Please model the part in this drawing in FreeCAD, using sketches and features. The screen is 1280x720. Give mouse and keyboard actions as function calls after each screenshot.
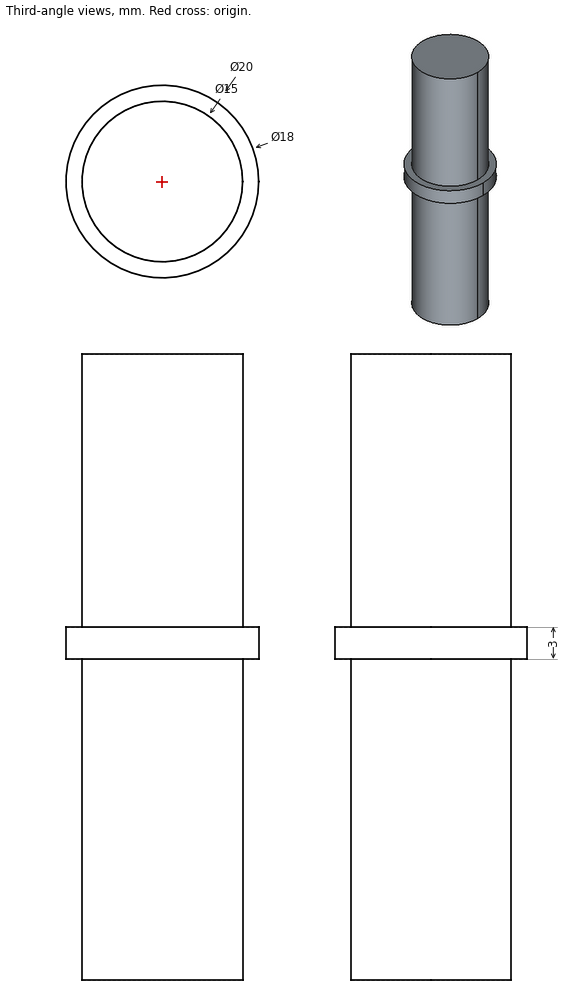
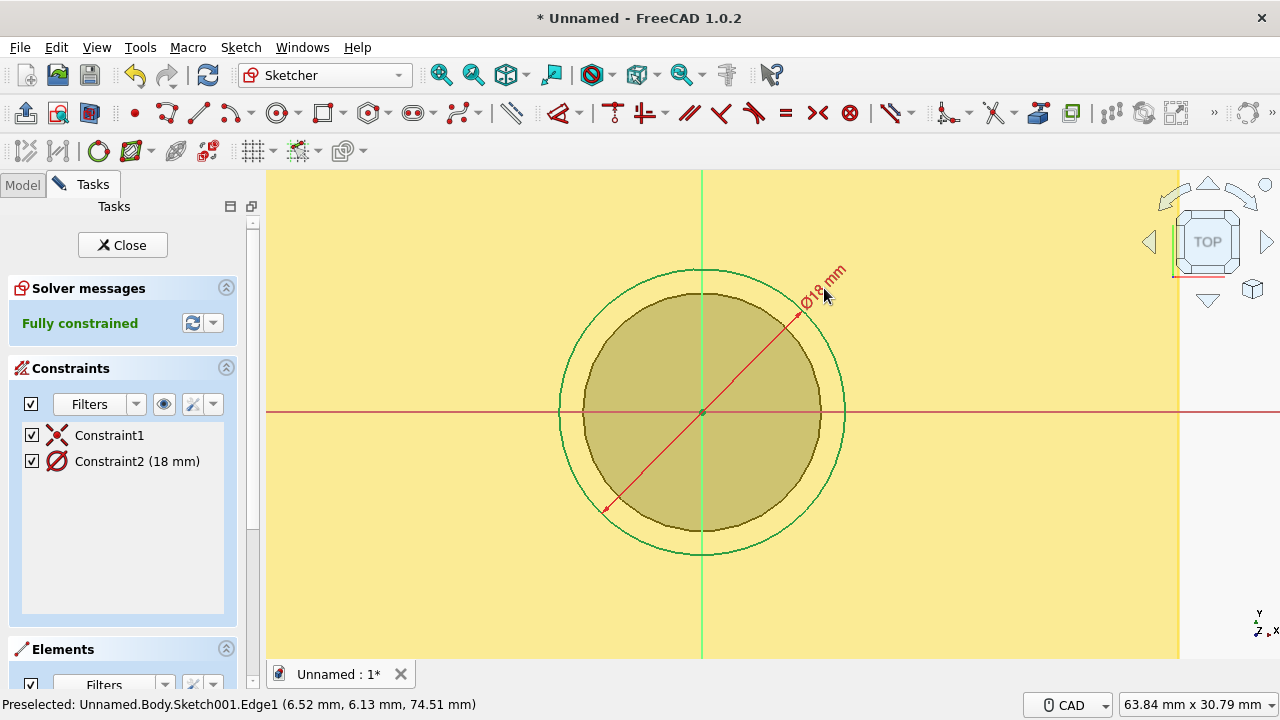
click(123, 245)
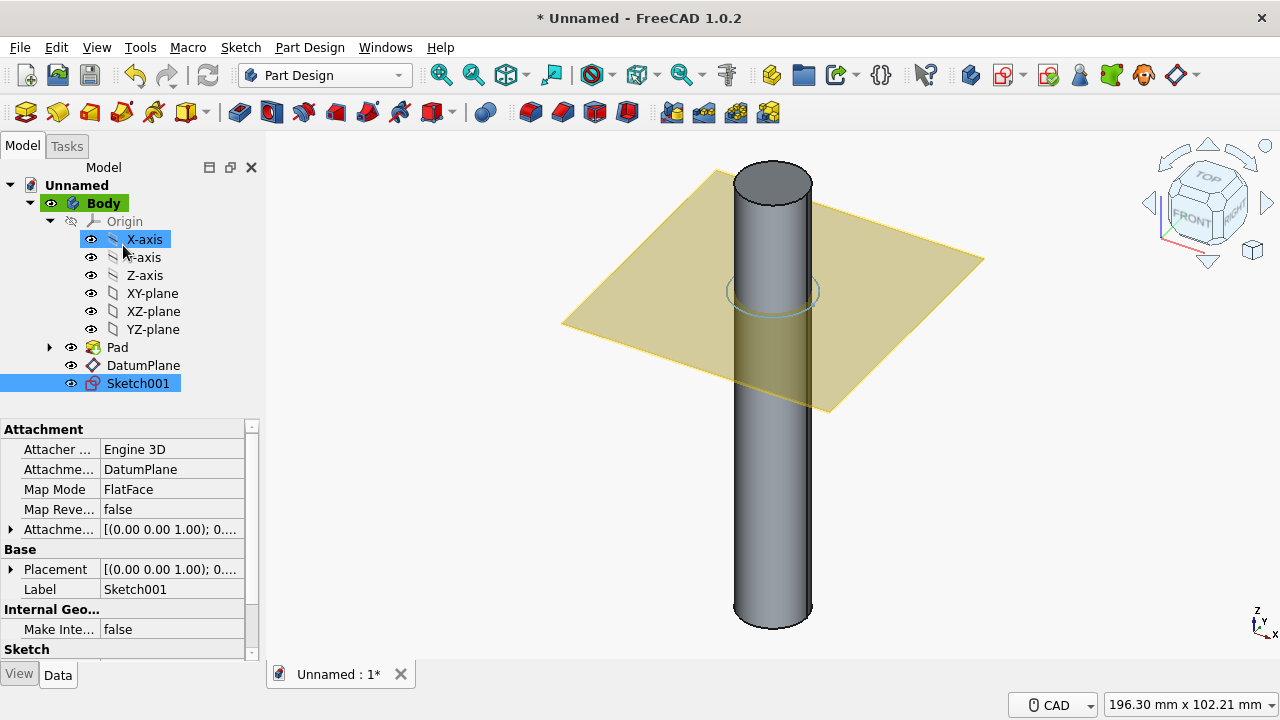
click(26, 112)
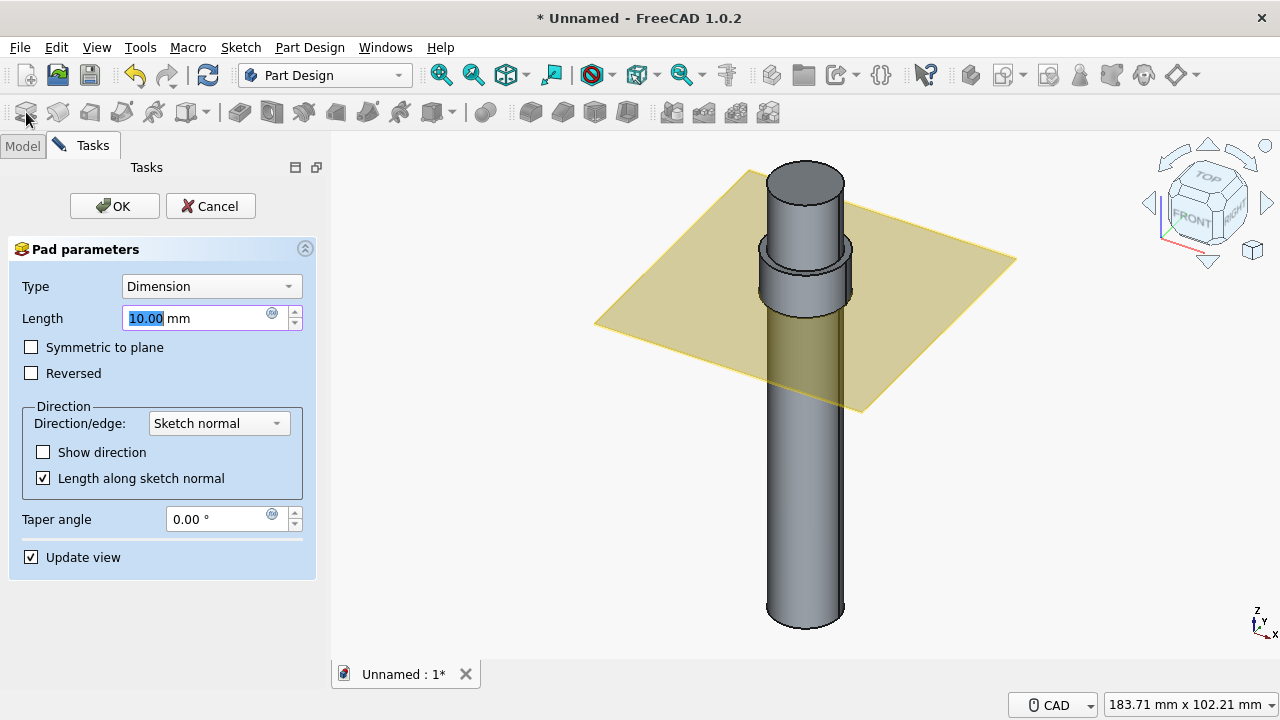
text(3)
key(Tab)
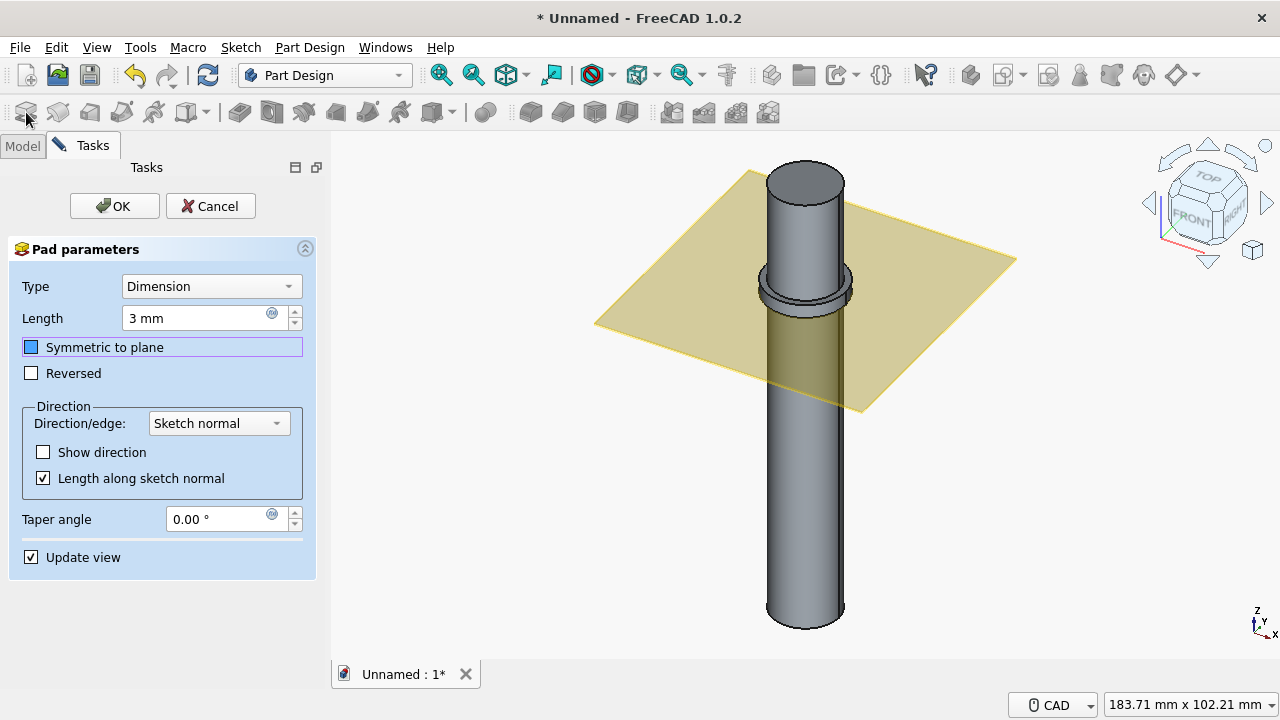
click(30, 373)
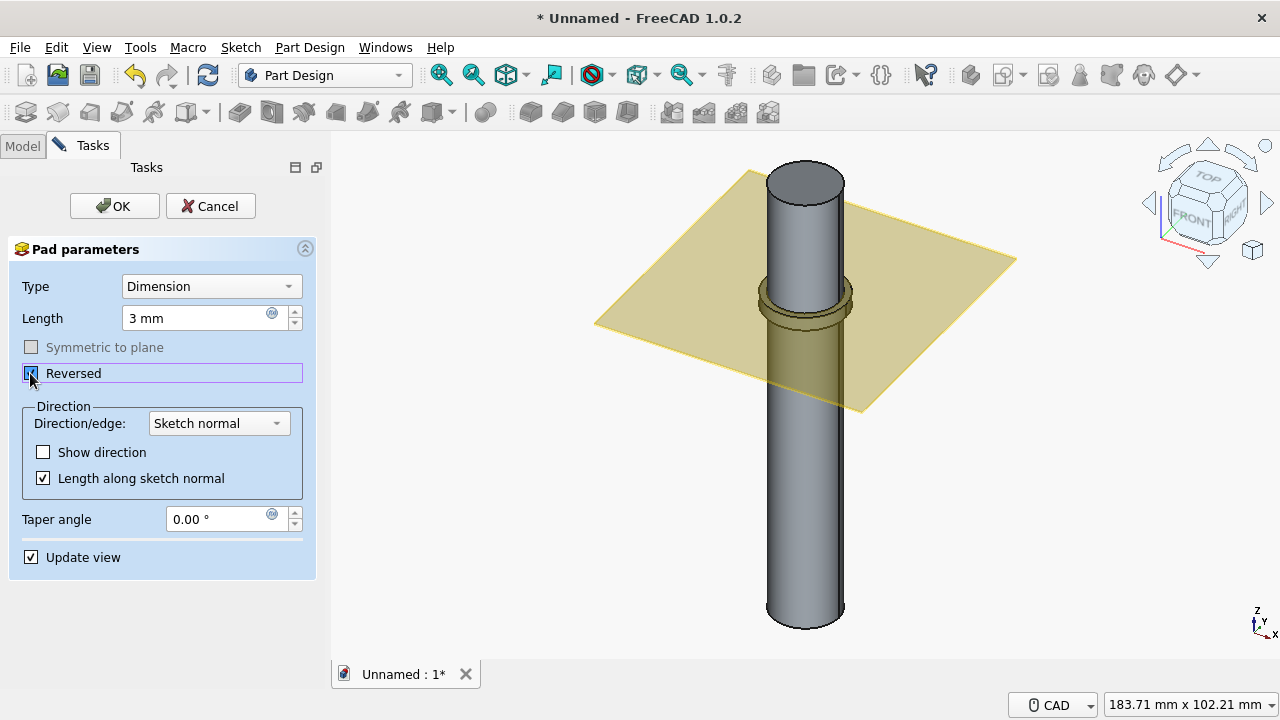
click(115, 206)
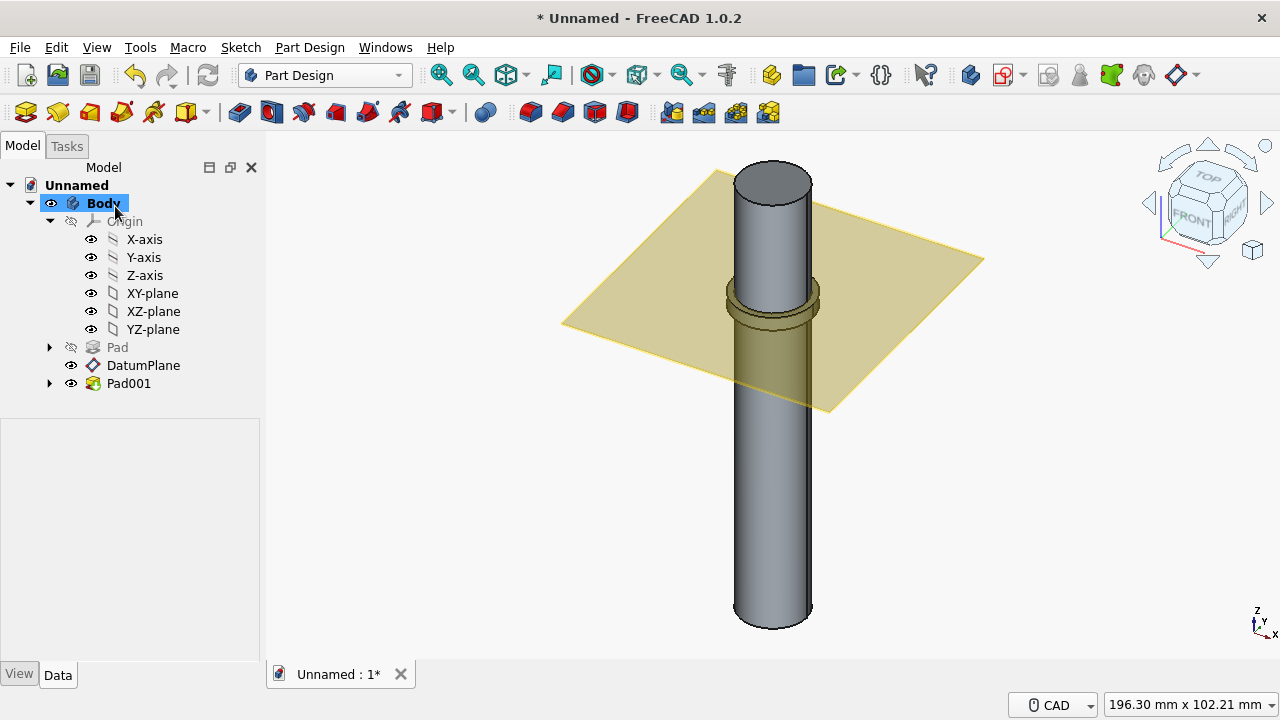
click(116, 365)
key(space)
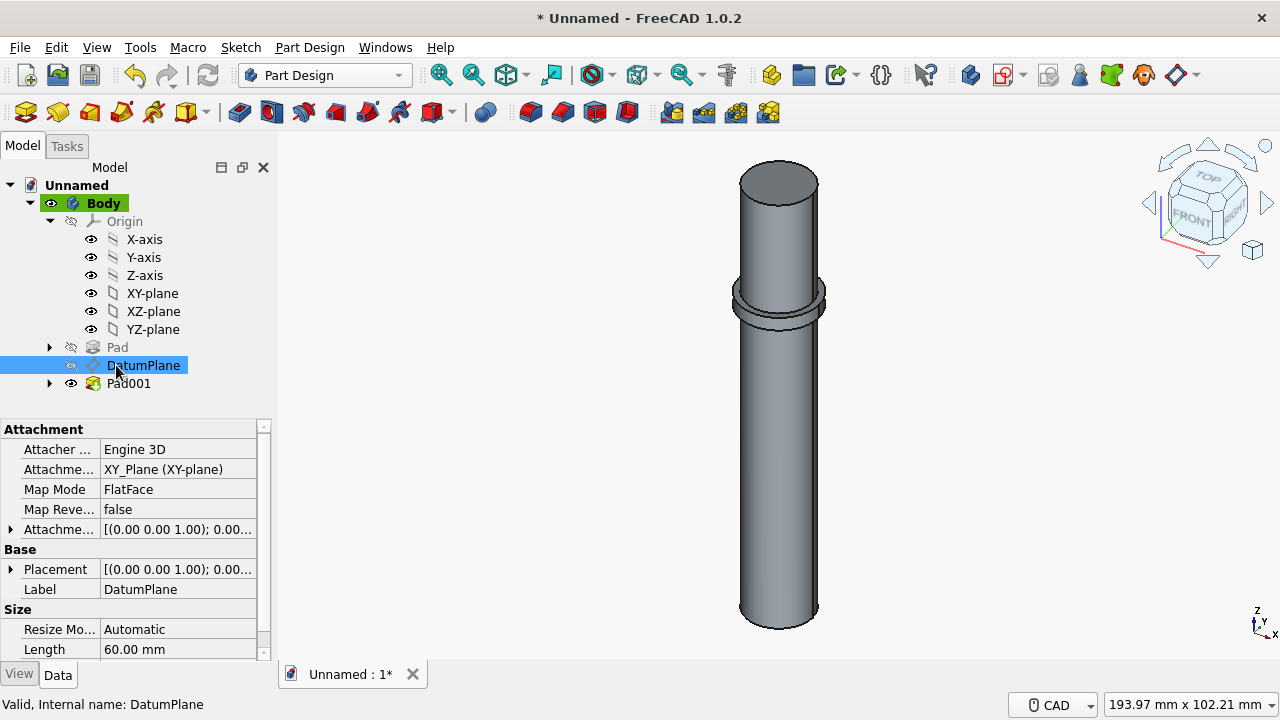
click(136, 293)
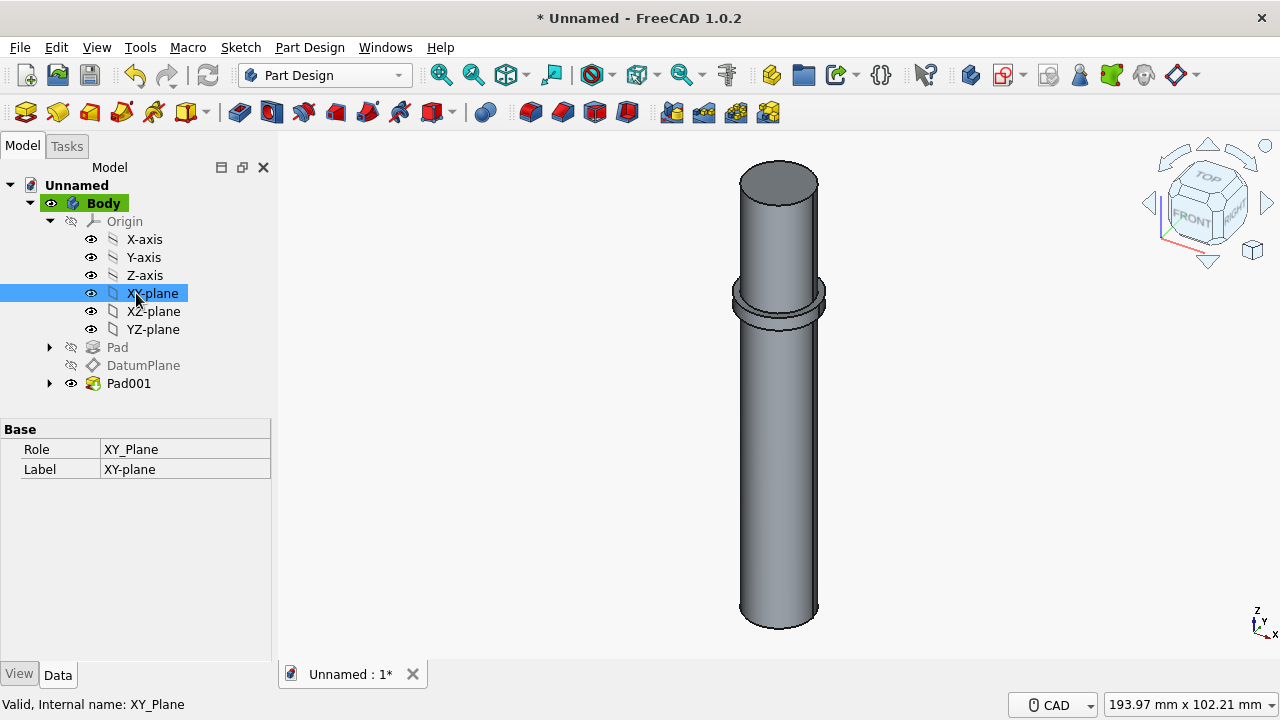
click(1176, 76)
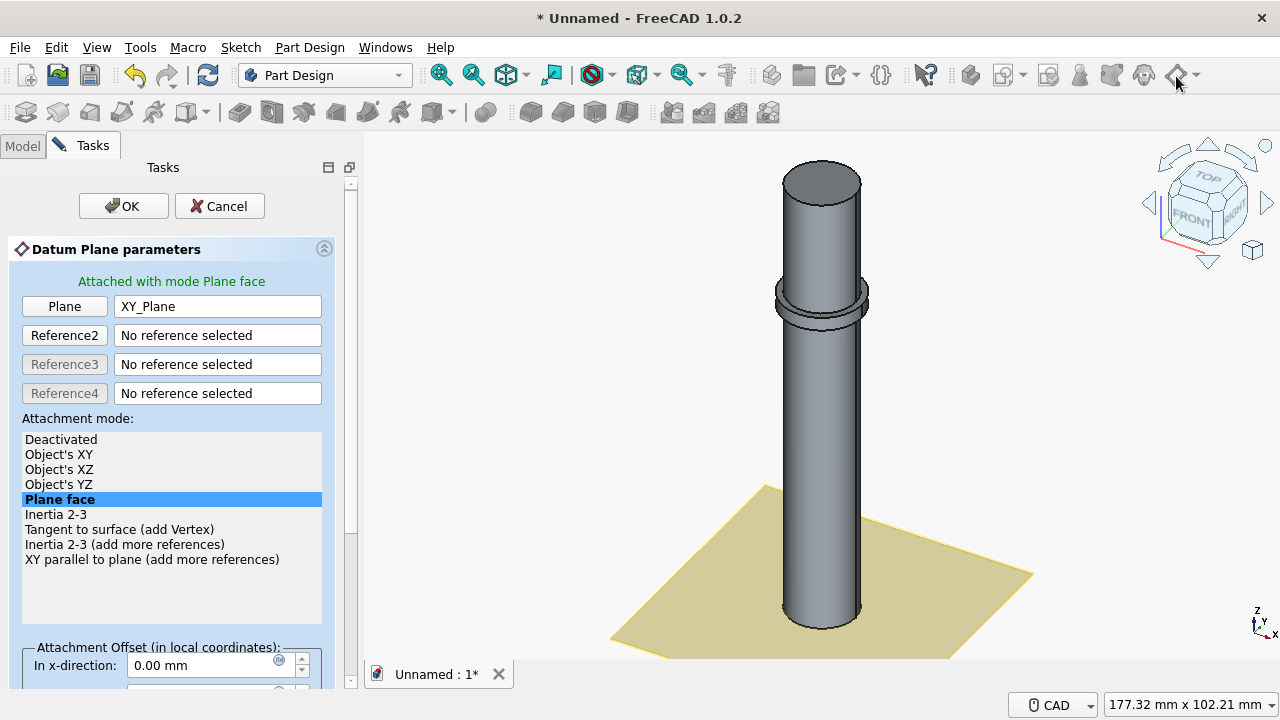
scroll(351, 432, down, 2)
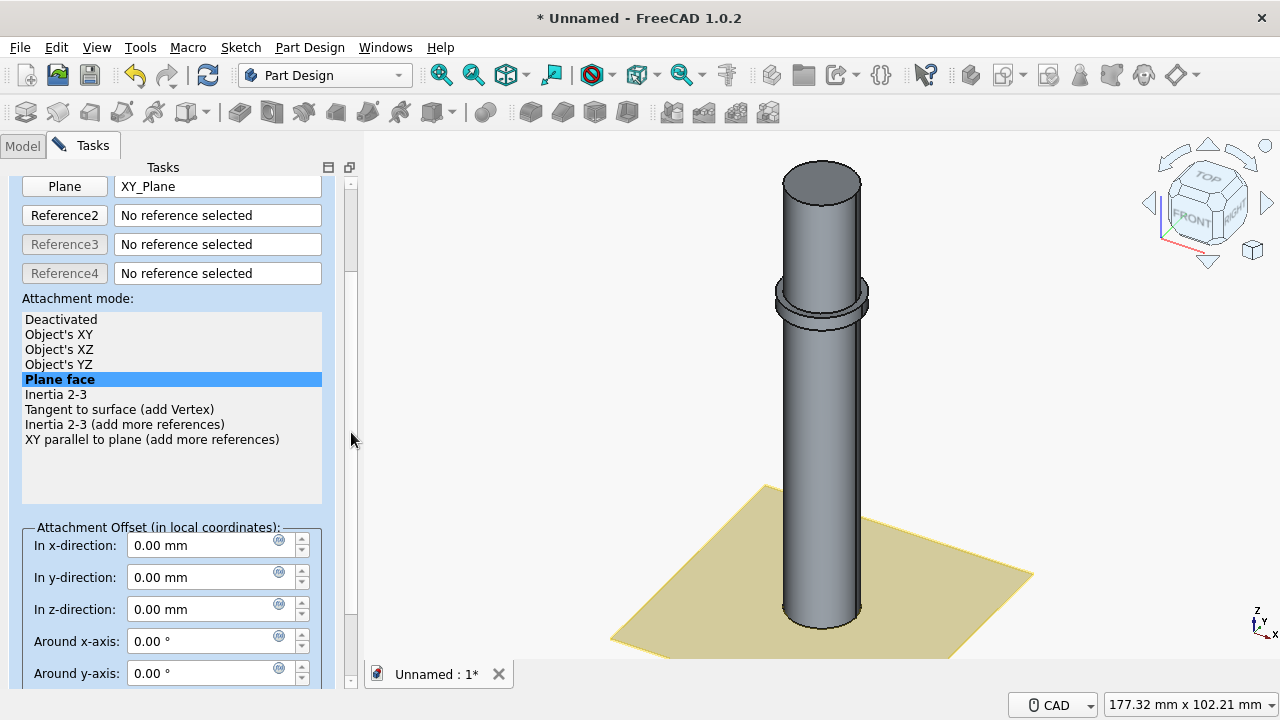
triple_click(210, 609)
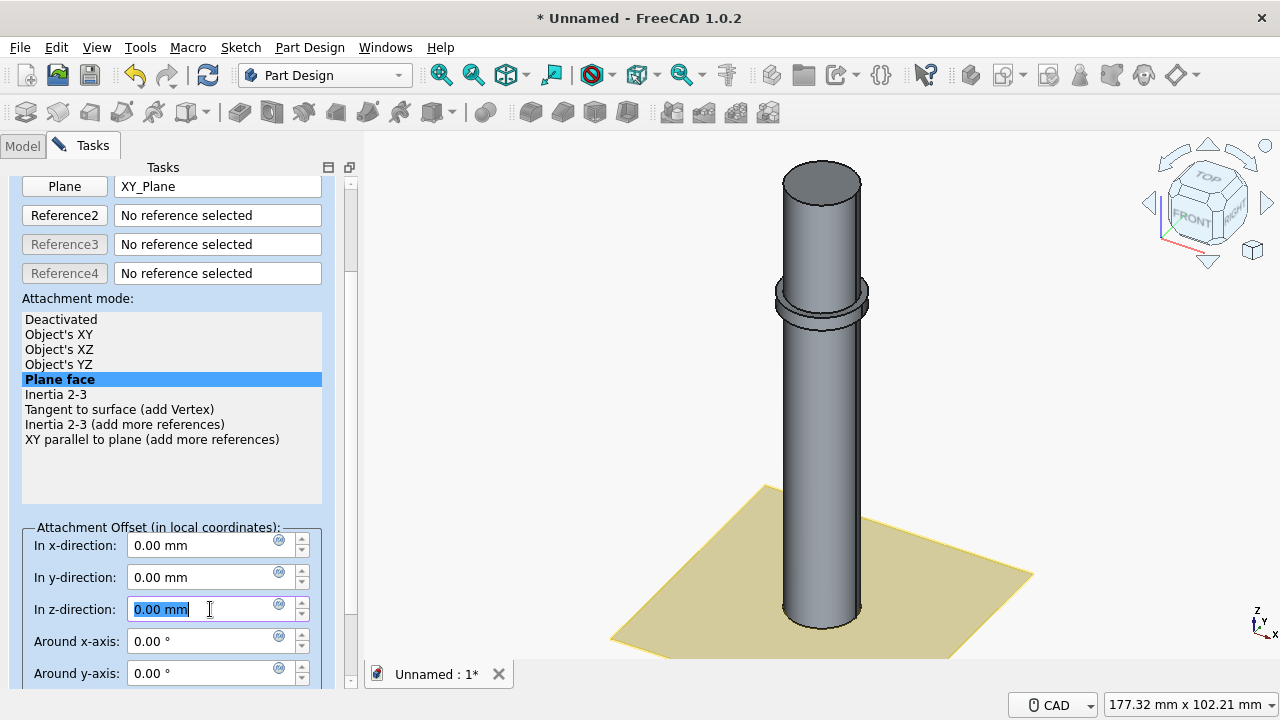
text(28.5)
key(Tab)